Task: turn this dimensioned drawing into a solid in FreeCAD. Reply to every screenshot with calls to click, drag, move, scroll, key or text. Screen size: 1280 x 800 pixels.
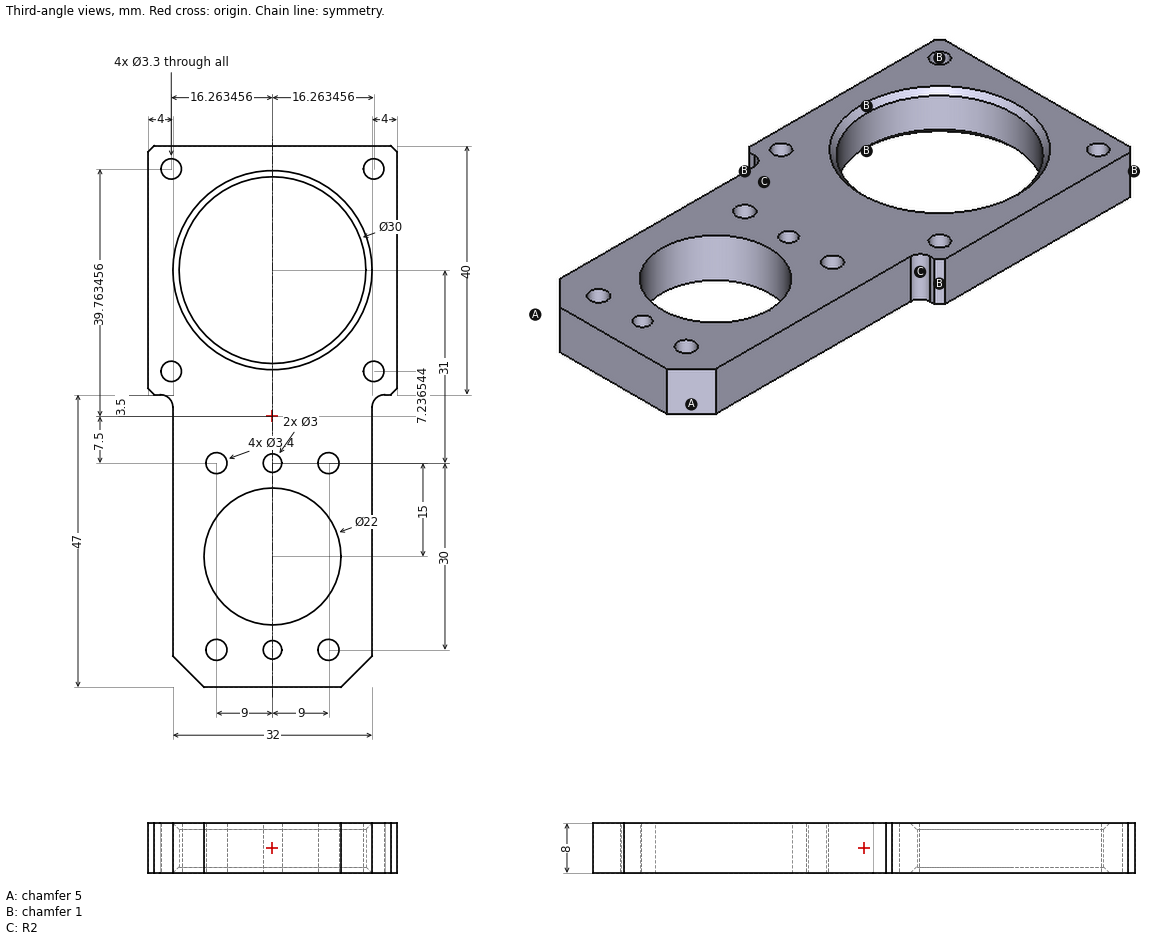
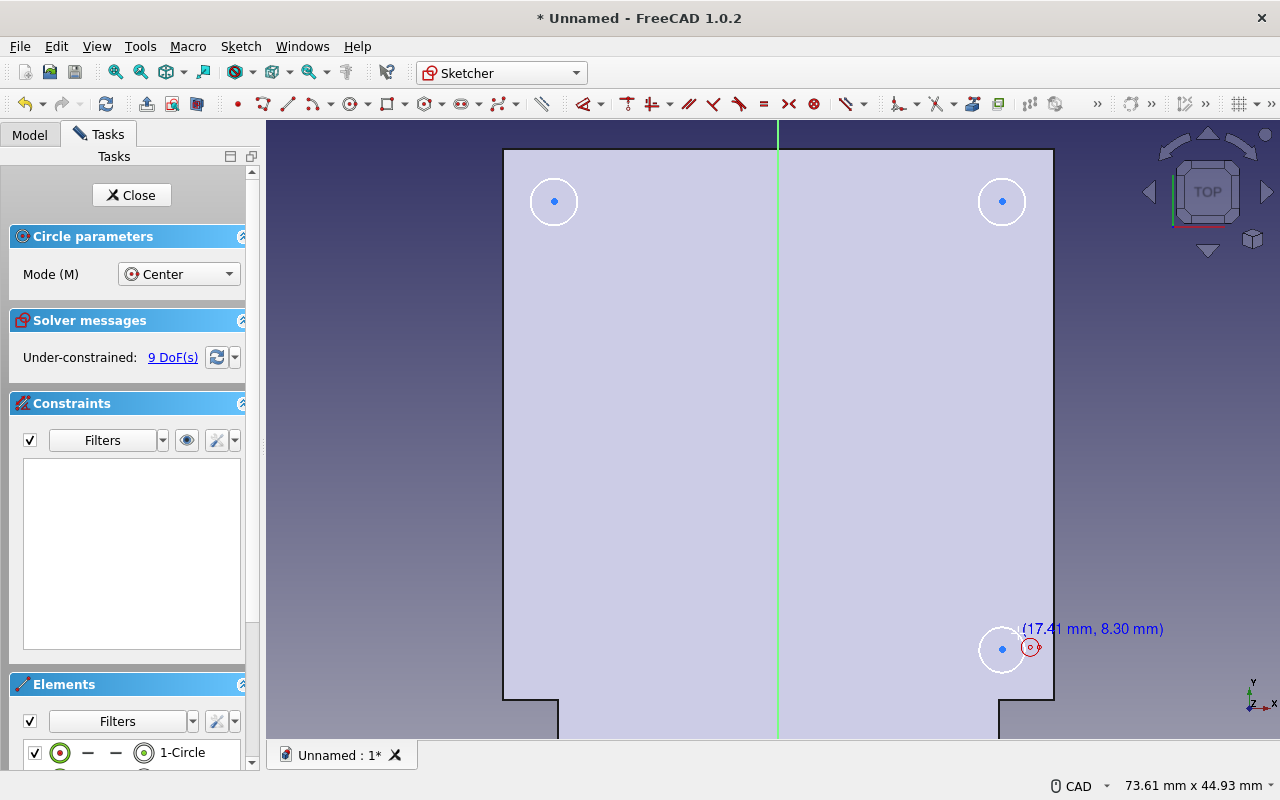
click(554, 649)
click(570, 633)
key(Escape)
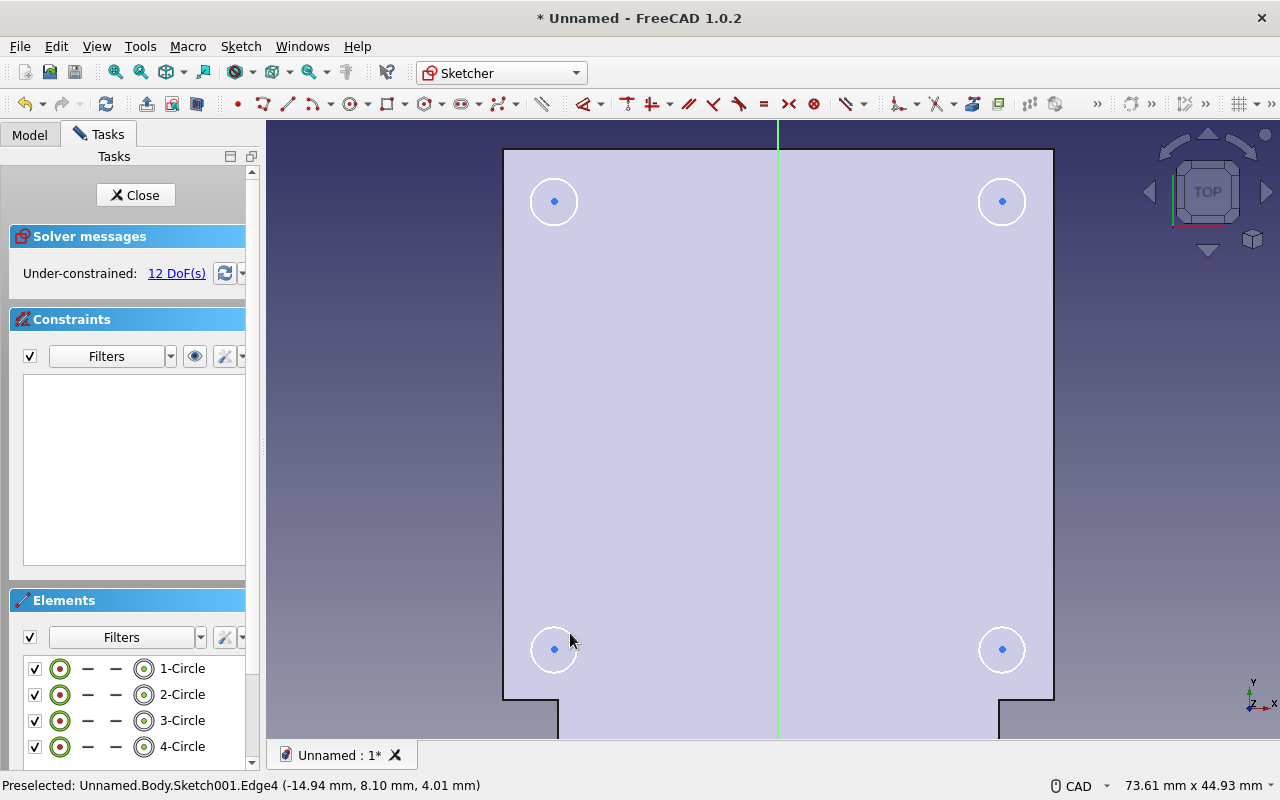
click(570, 185)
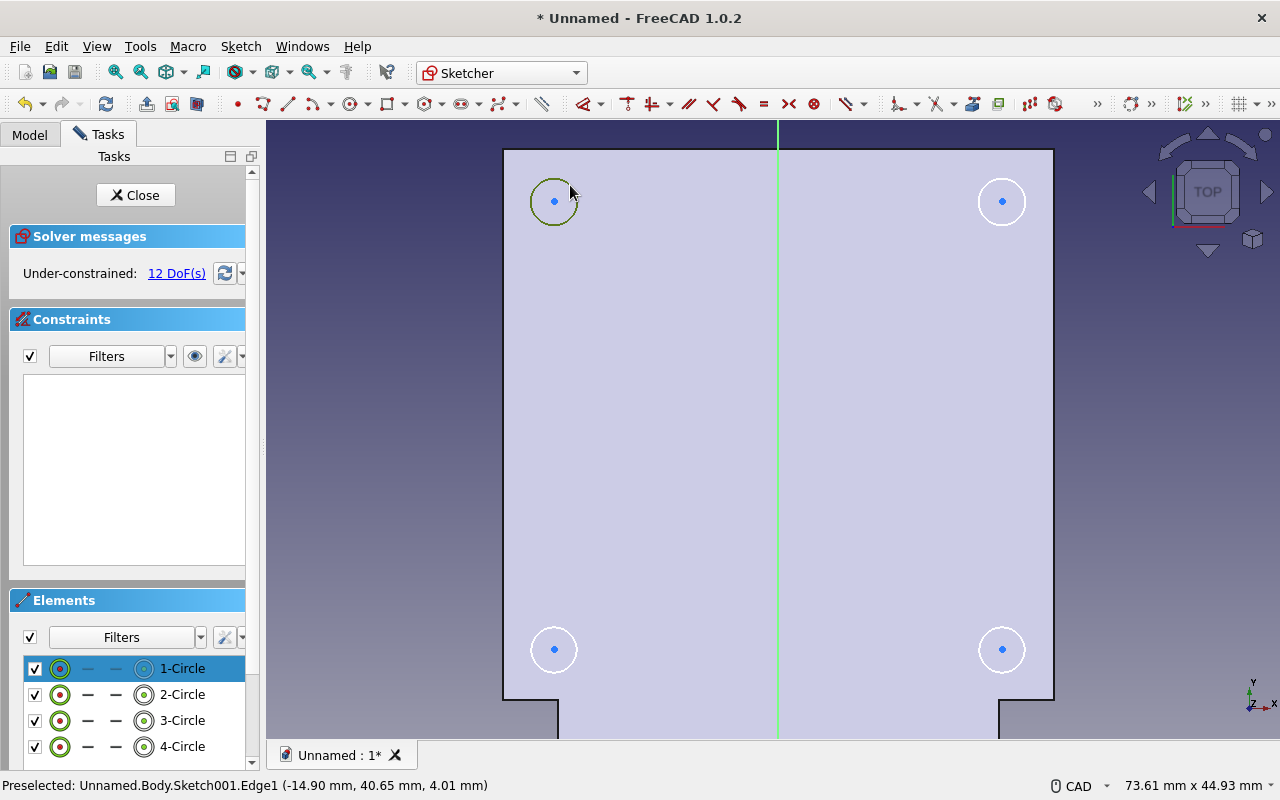
click(1018, 185)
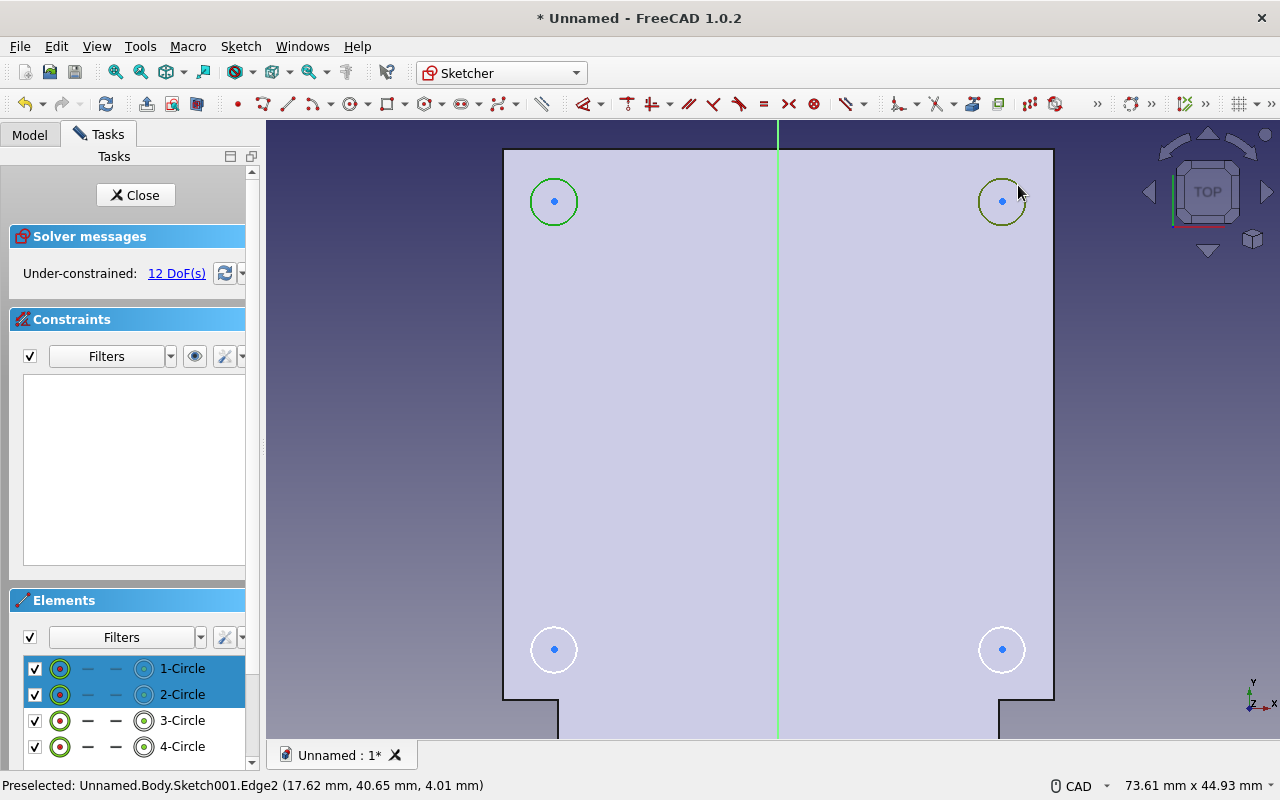
click(1018, 634)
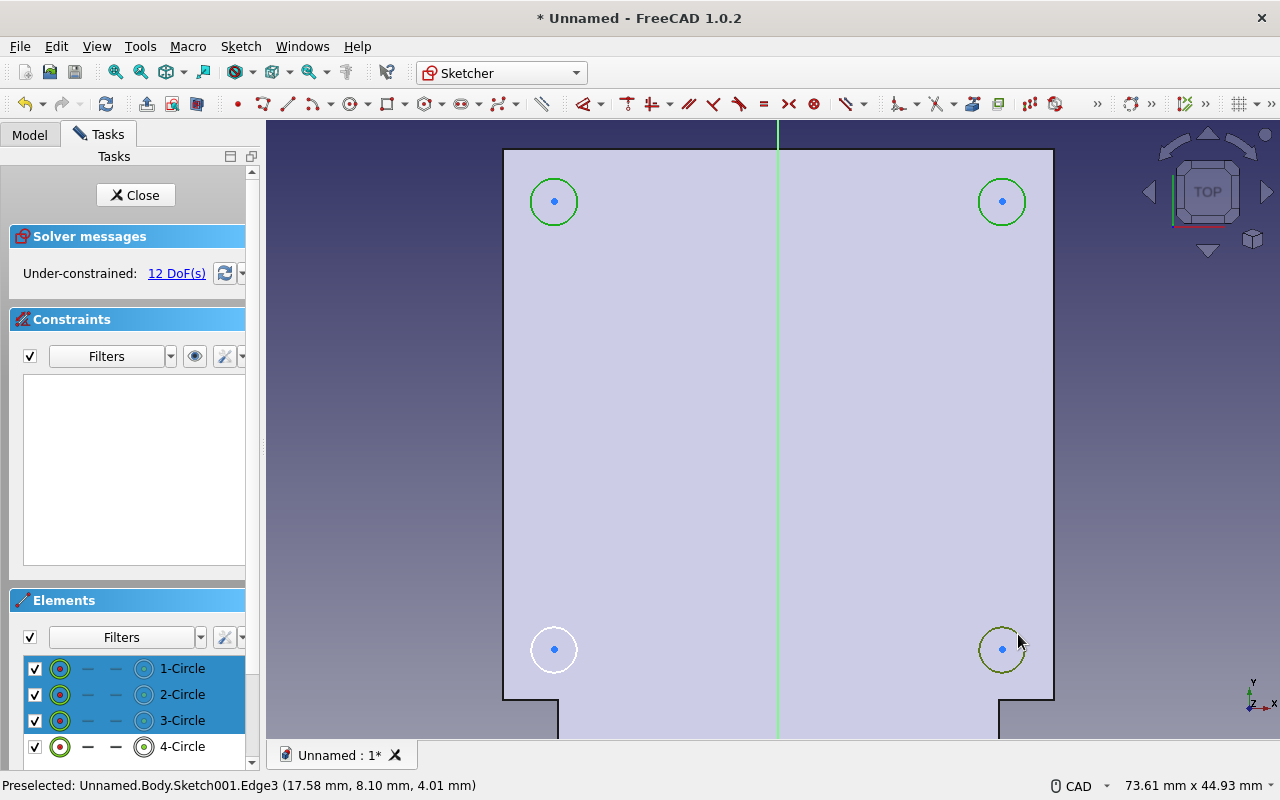
click(570, 634)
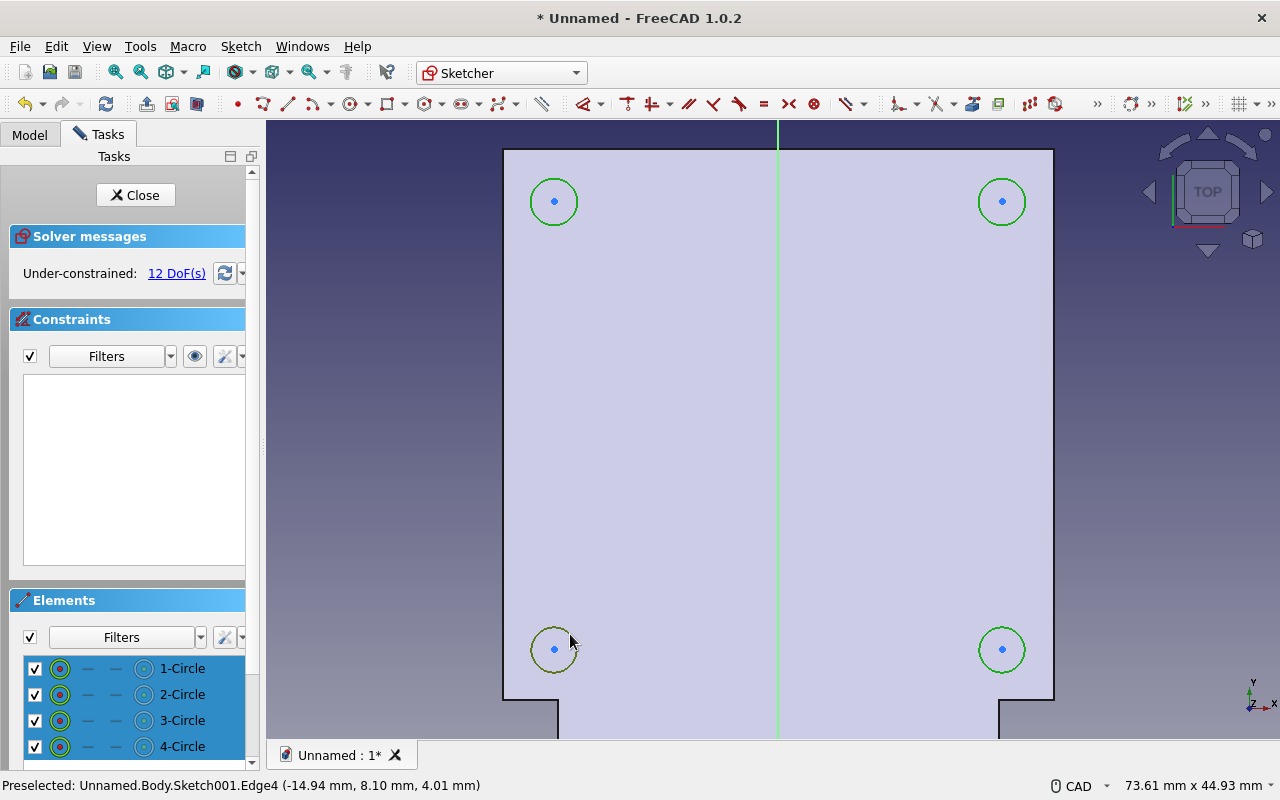
key(e)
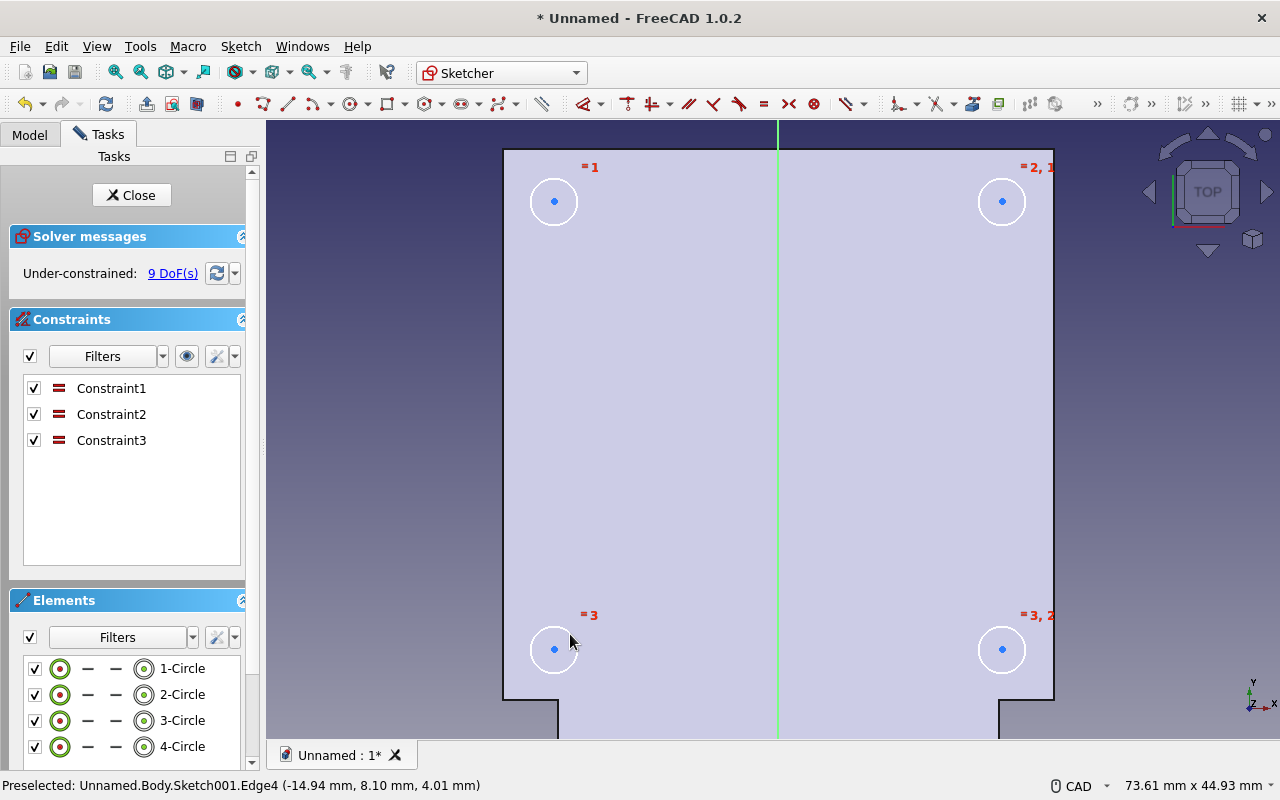
click(554, 202)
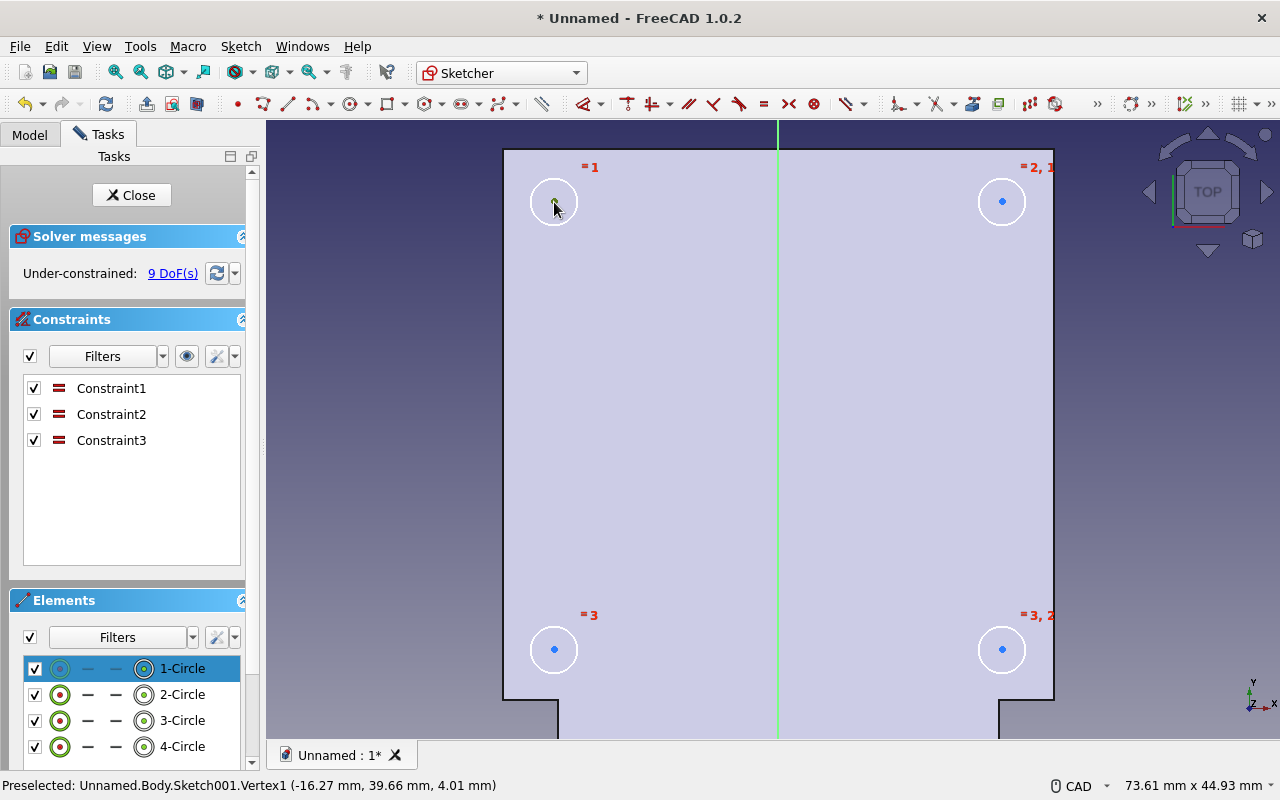
click(1002, 202)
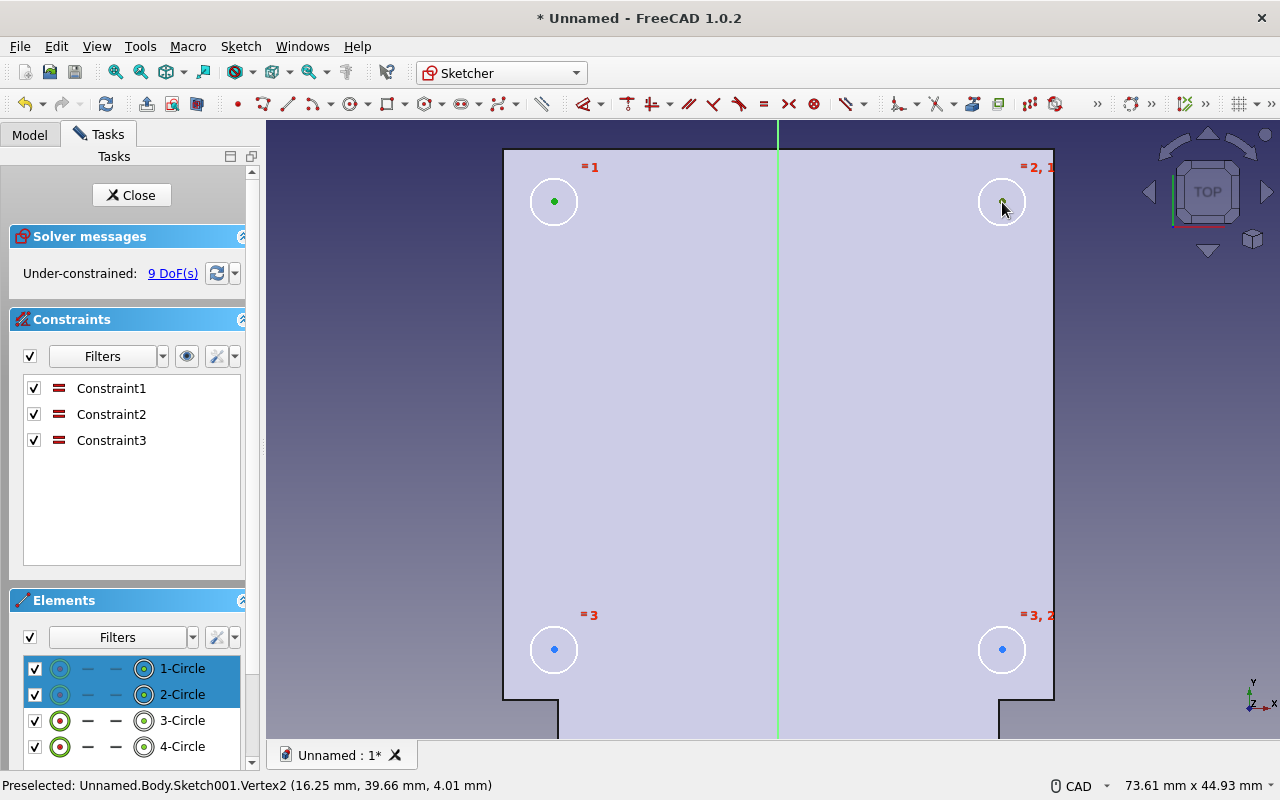
key(h)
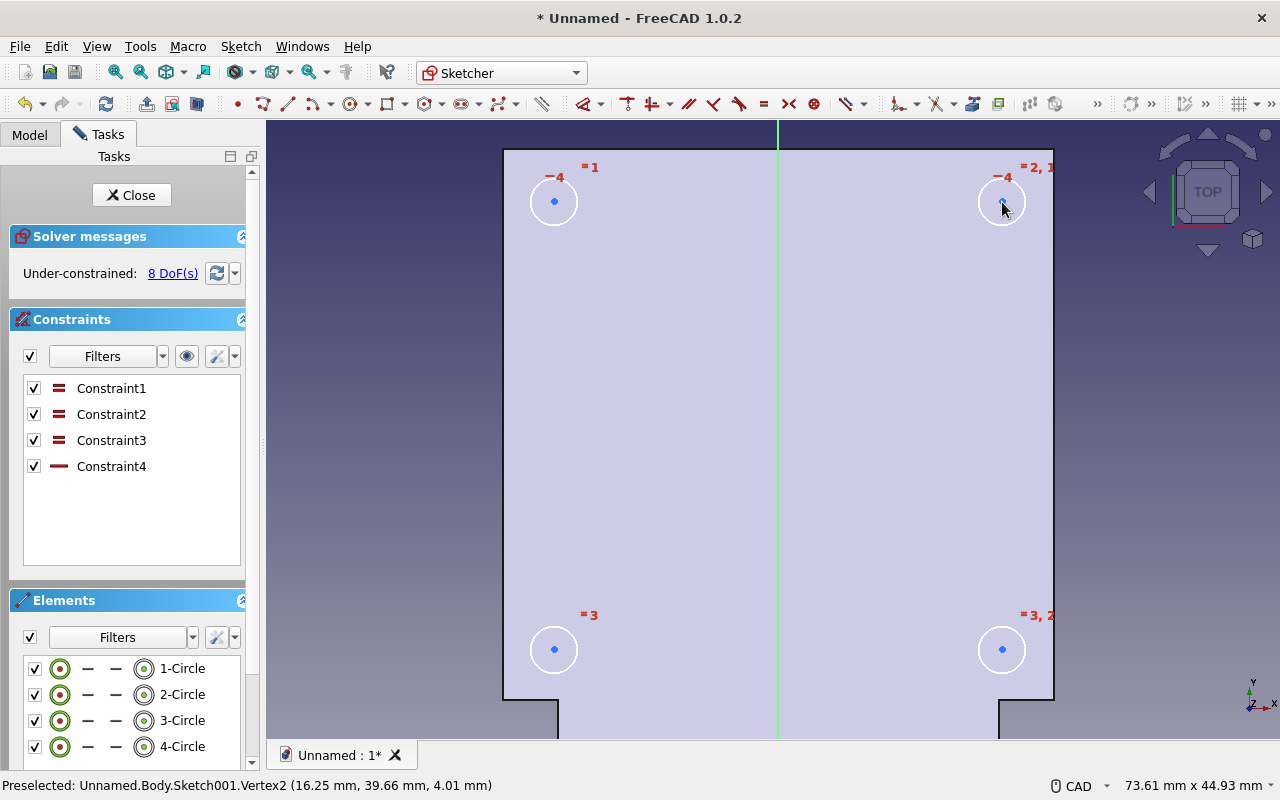
click(1002, 202)